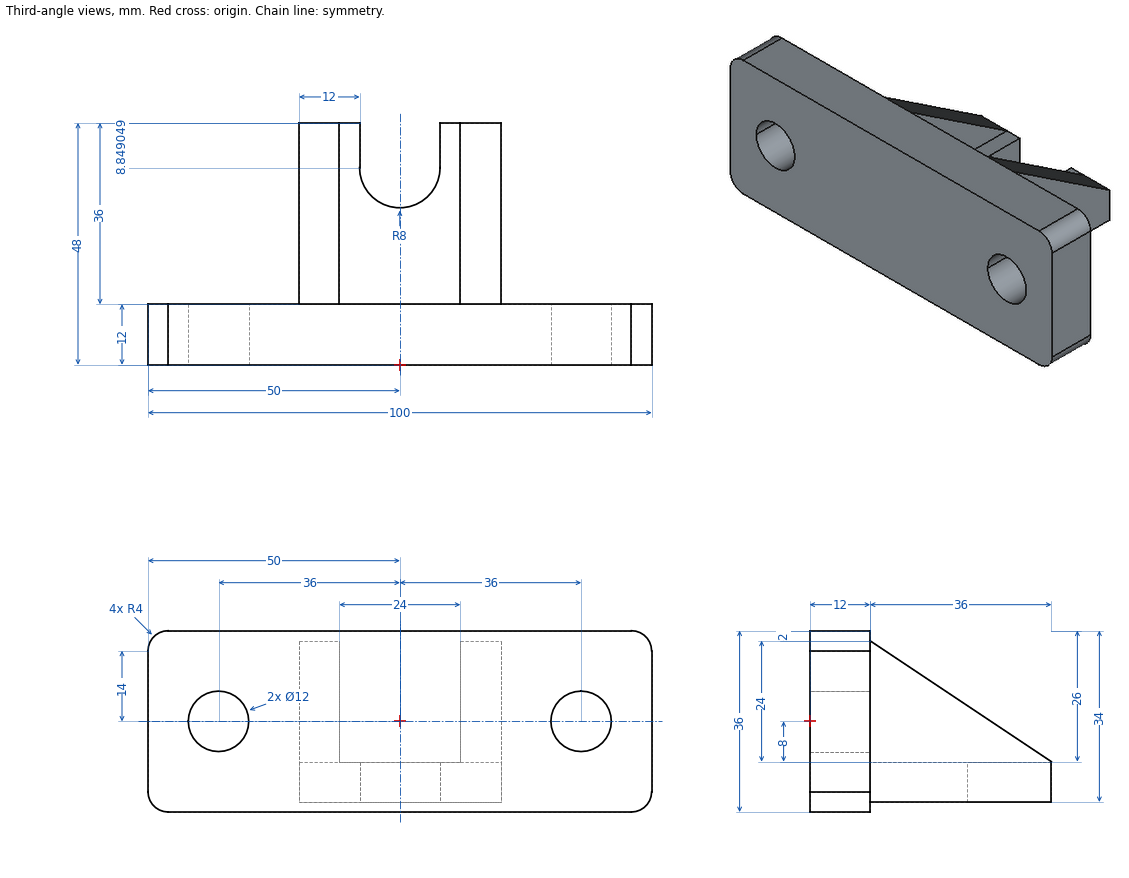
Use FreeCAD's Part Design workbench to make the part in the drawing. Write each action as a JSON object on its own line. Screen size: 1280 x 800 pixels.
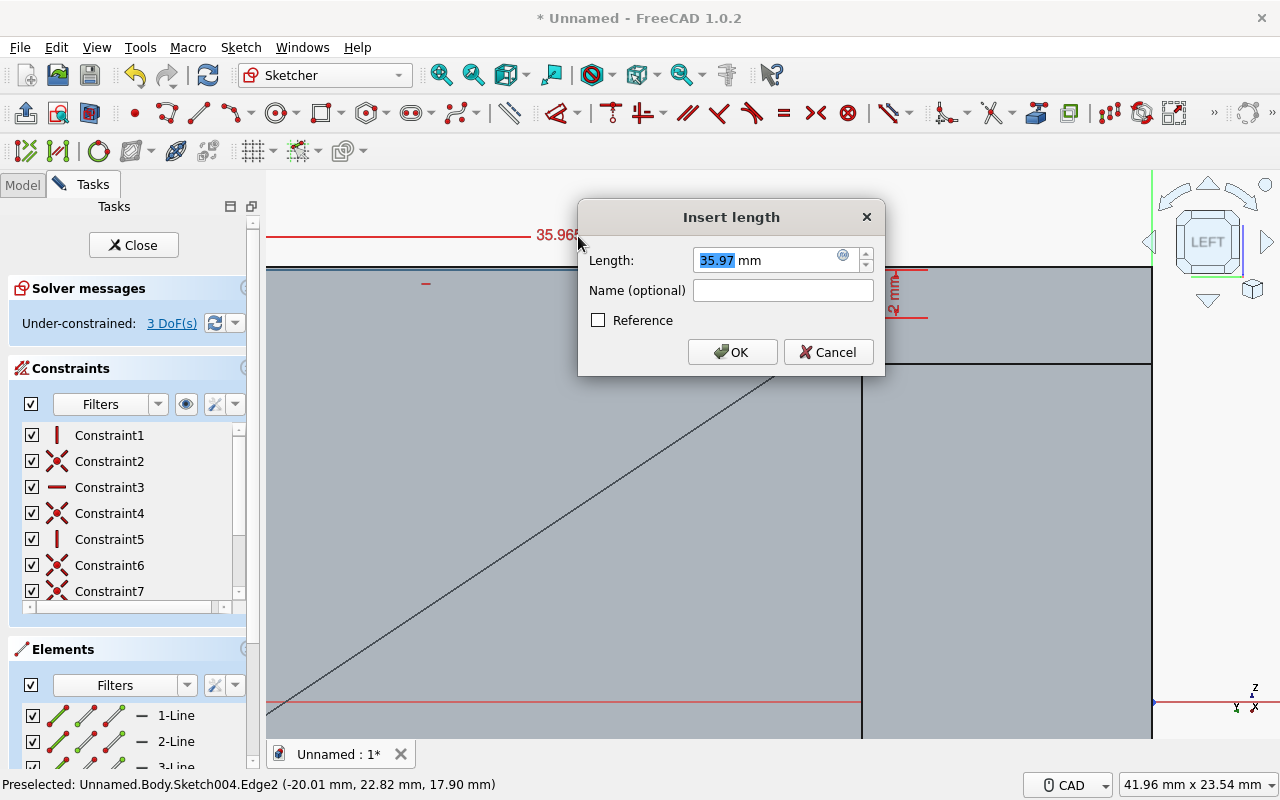
{"action": "type", "text": "36"}
{"action": "key", "text": "Return"}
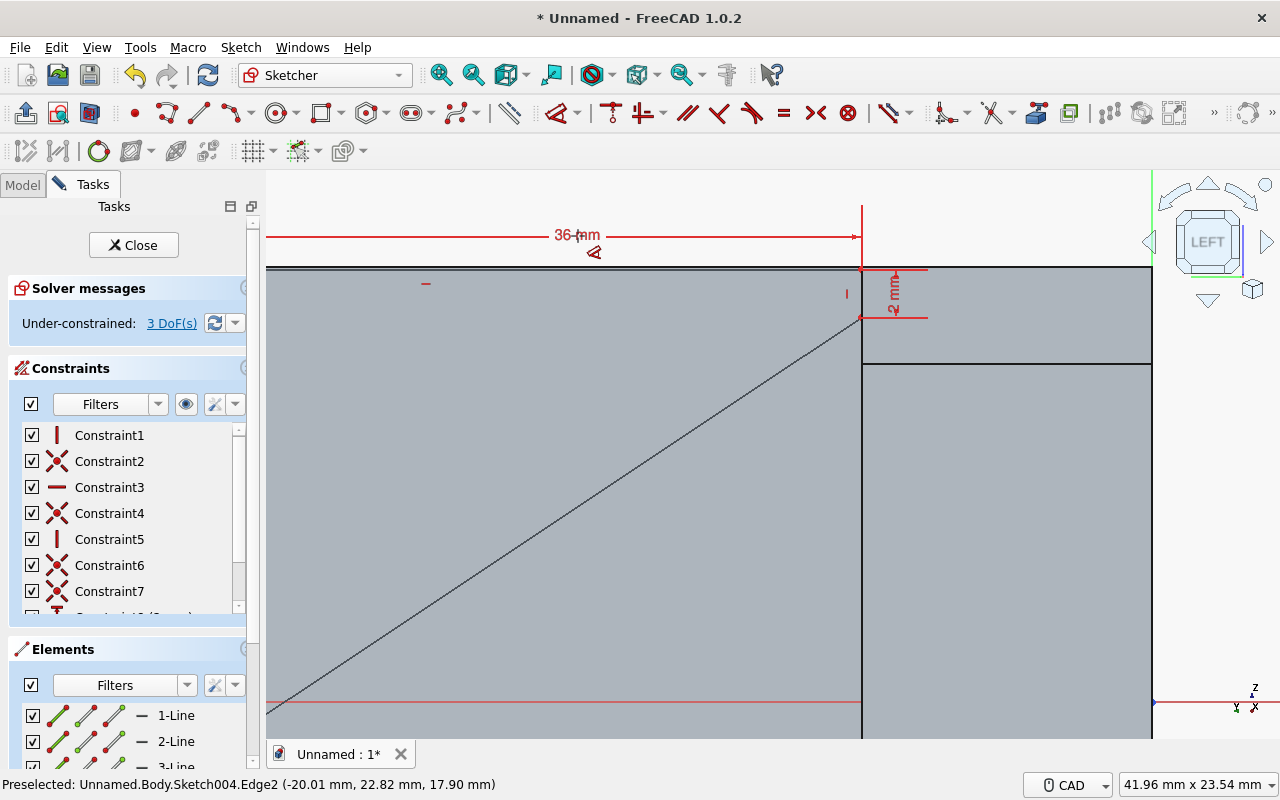
{"action": "scroll", "coordinate": [865, 300], "scroll_direction": "down", "scroll_amount": 3}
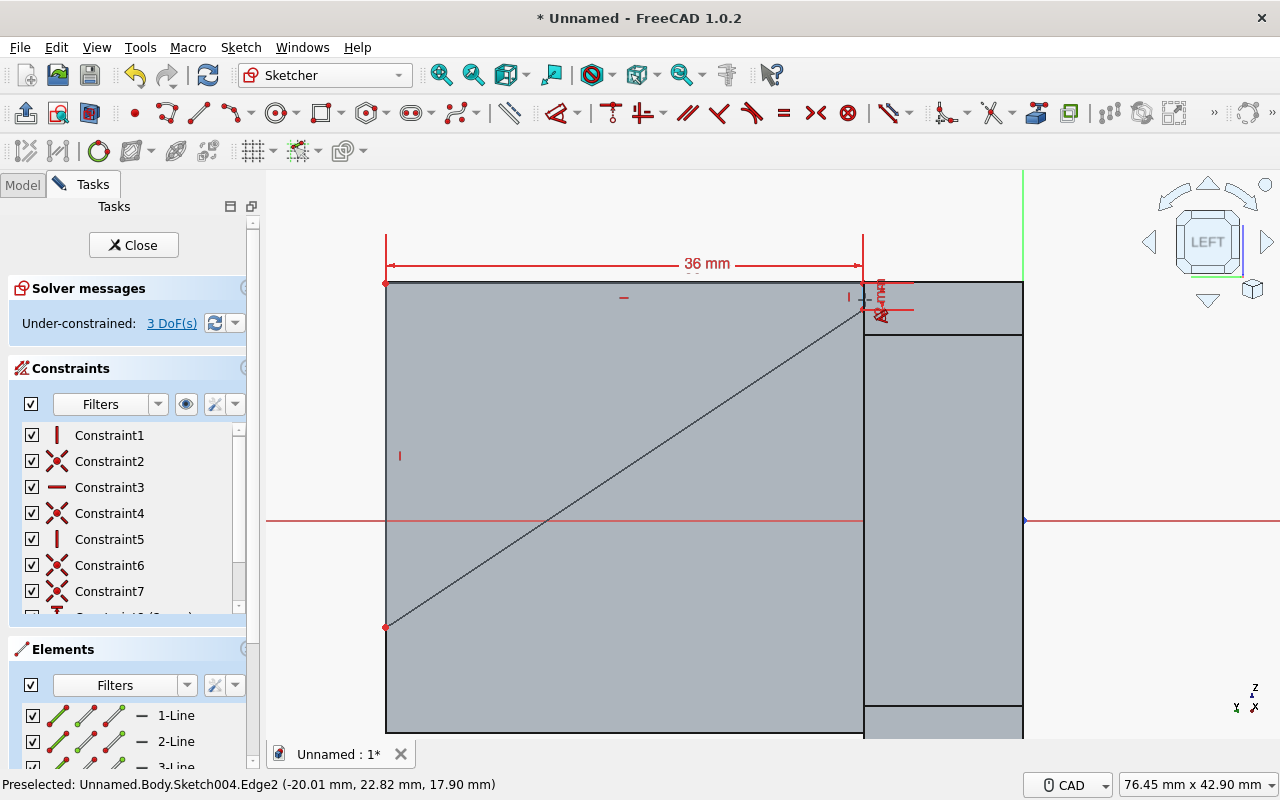
{"action": "left_click", "coordinate": [386, 387]}
{"action": "left_click", "coordinate": [352, 456]}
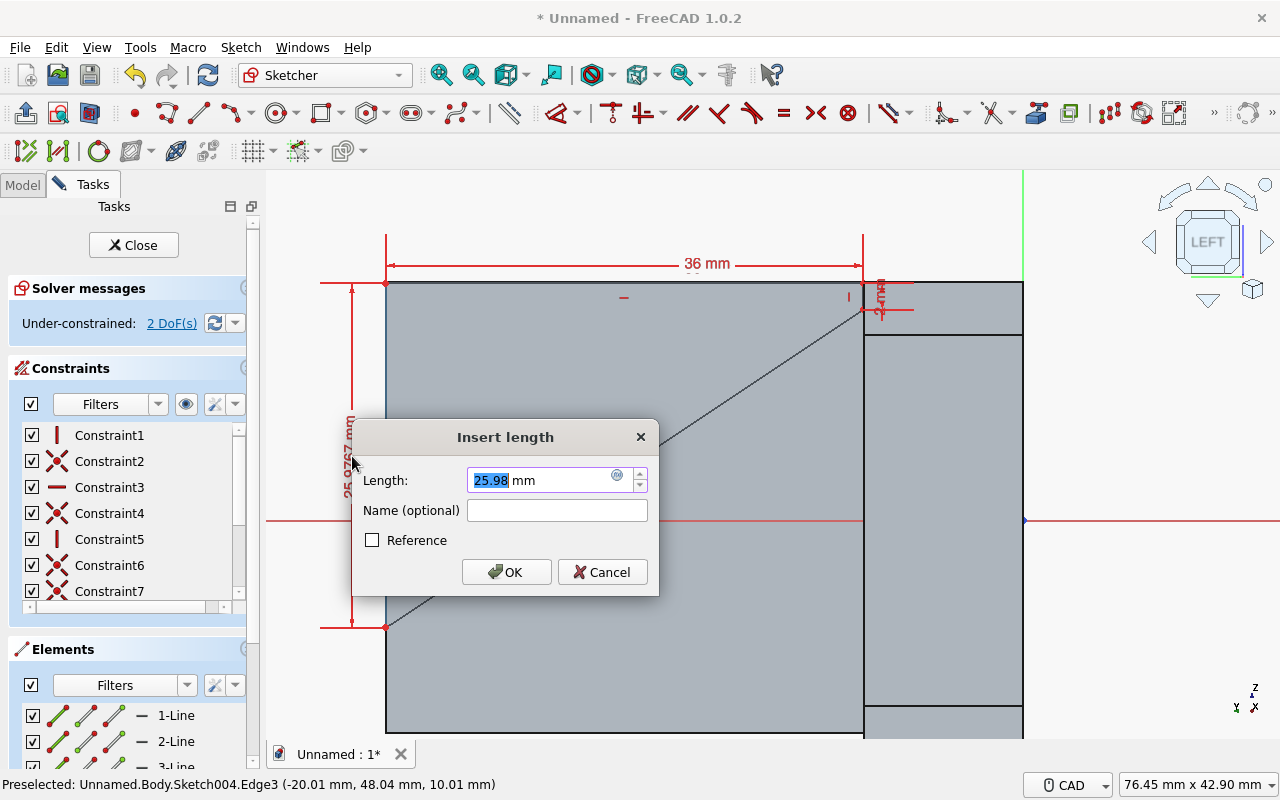
{"action": "type", "text": "26"}
{"action": "key", "text": "Return"}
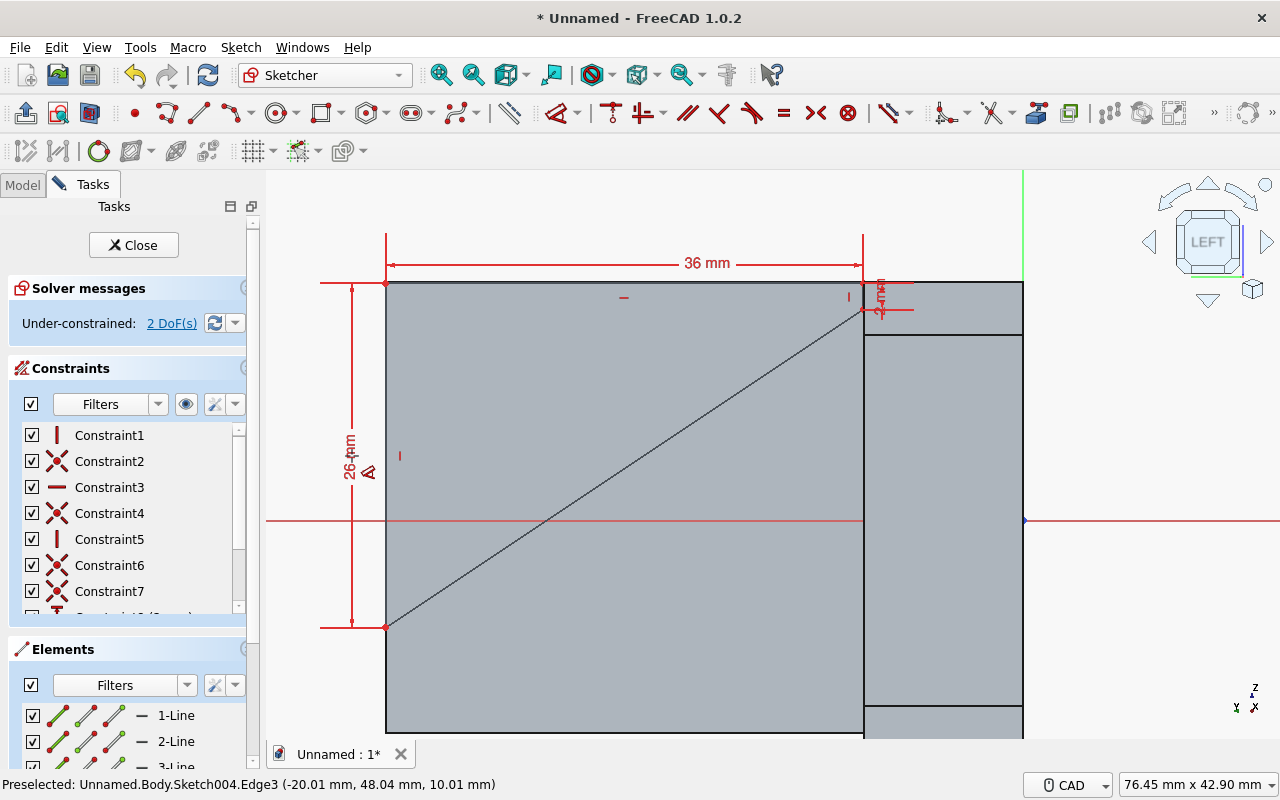
{"action": "left_click", "coordinate": [386, 628]}
{"action": "left_click", "coordinate": [352, 574]}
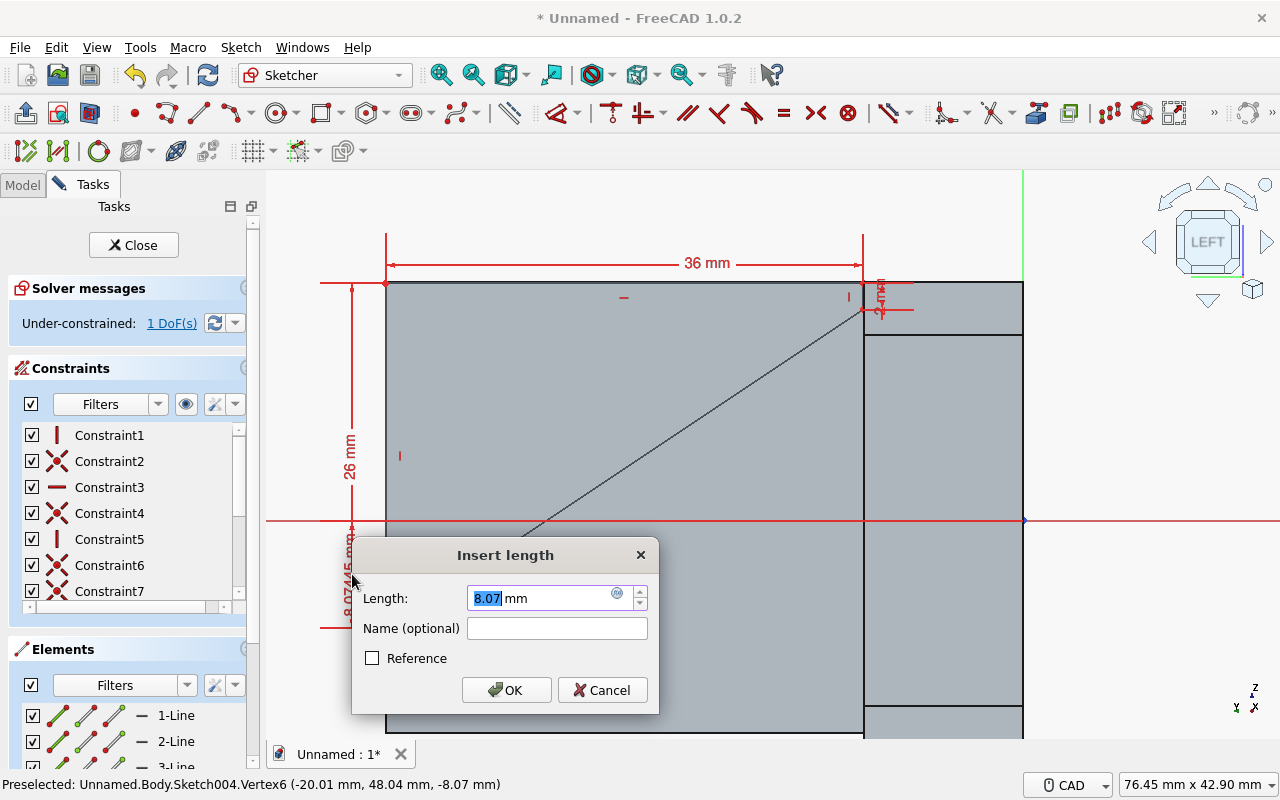
{"action": "type", "text": "8"}
{"action": "key", "text": "Return"}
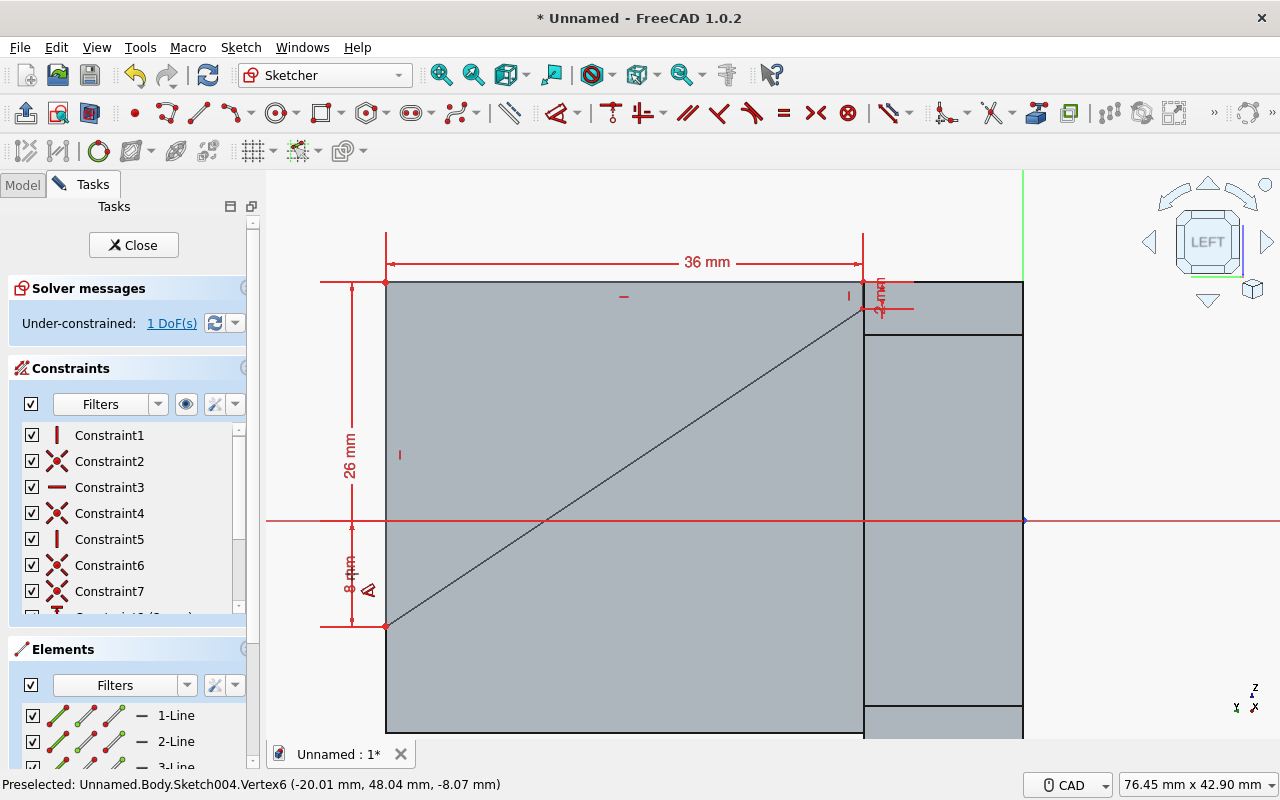
{"action": "left_click", "coordinate": [863, 309]}
{"action": "left_click", "coordinate": [943, 275]}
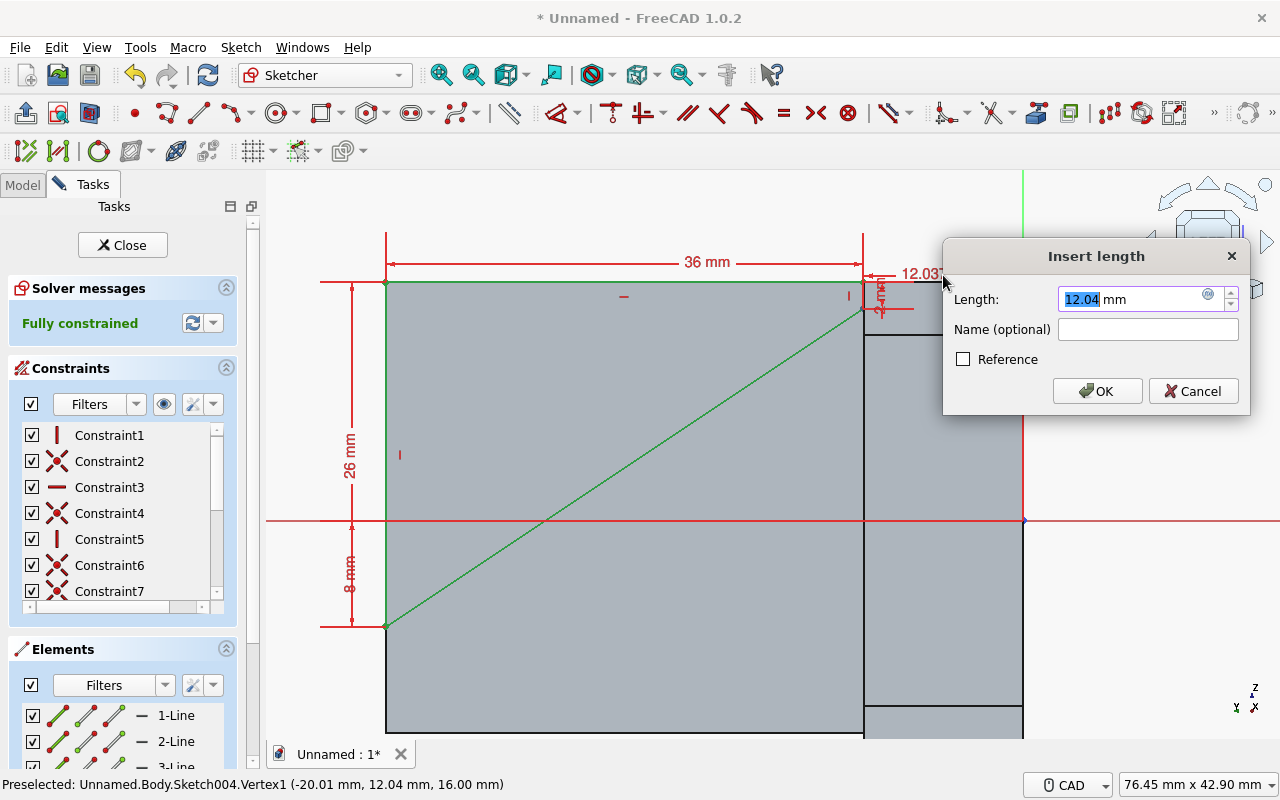
{"action": "type", "text": "12"}
{"action": "key", "text": "Return"}
{"action": "key", "text": "Escape"}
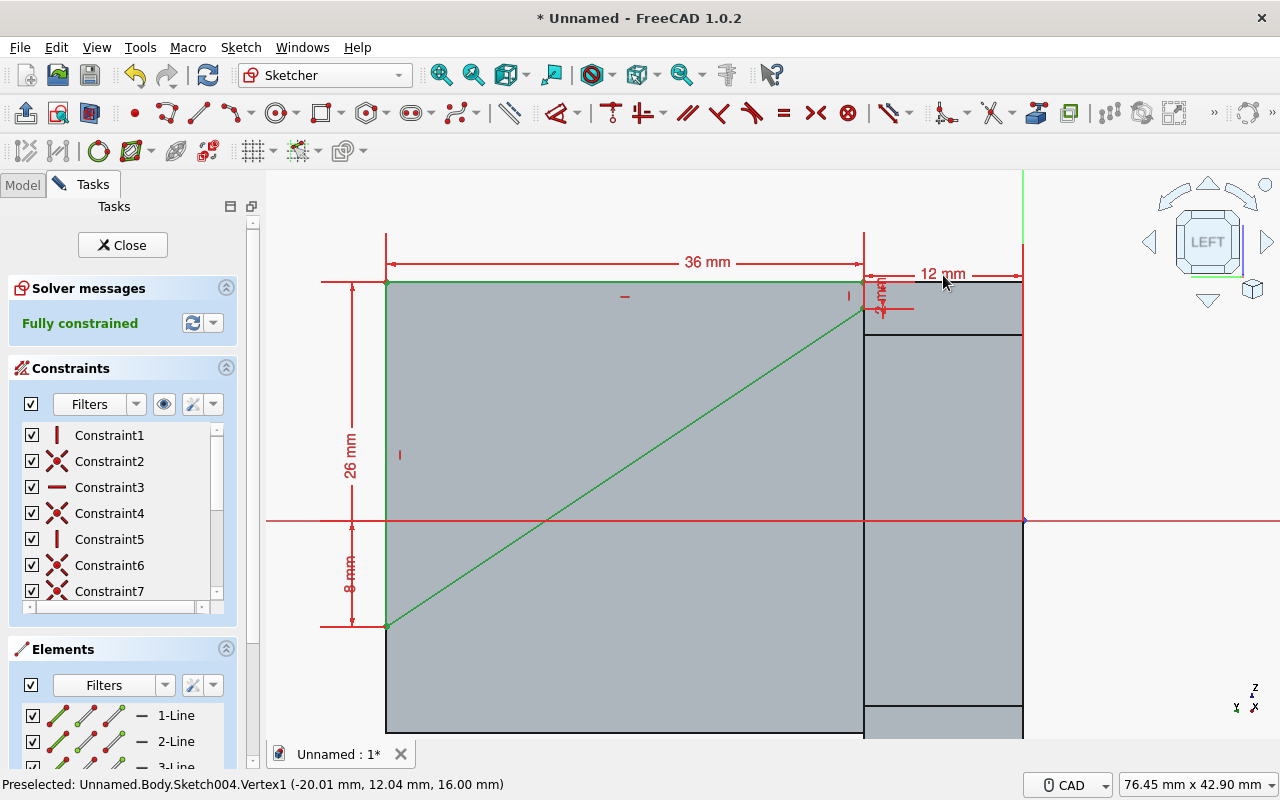
{"action": "left_click", "coordinate": [123, 245]}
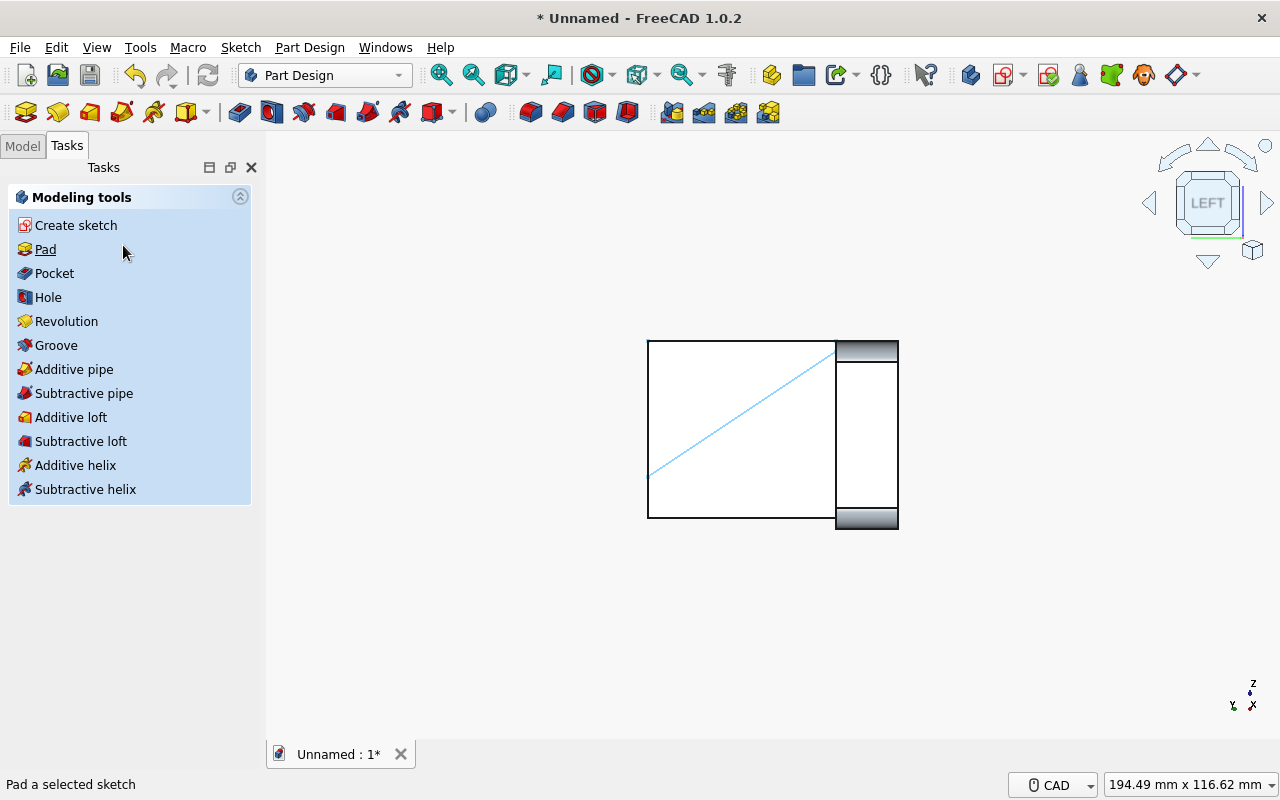
{"action": "left_click", "coordinate": [240, 112]}